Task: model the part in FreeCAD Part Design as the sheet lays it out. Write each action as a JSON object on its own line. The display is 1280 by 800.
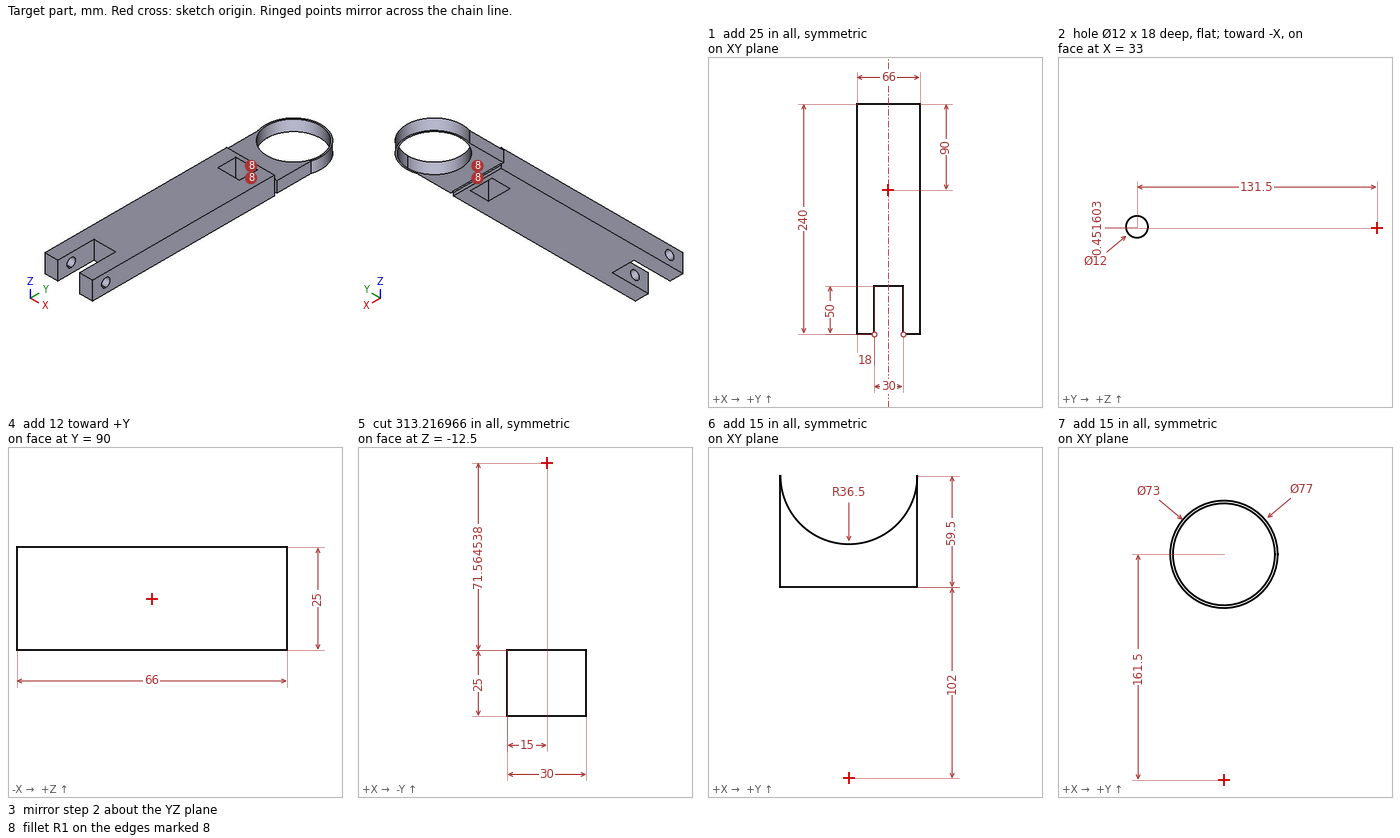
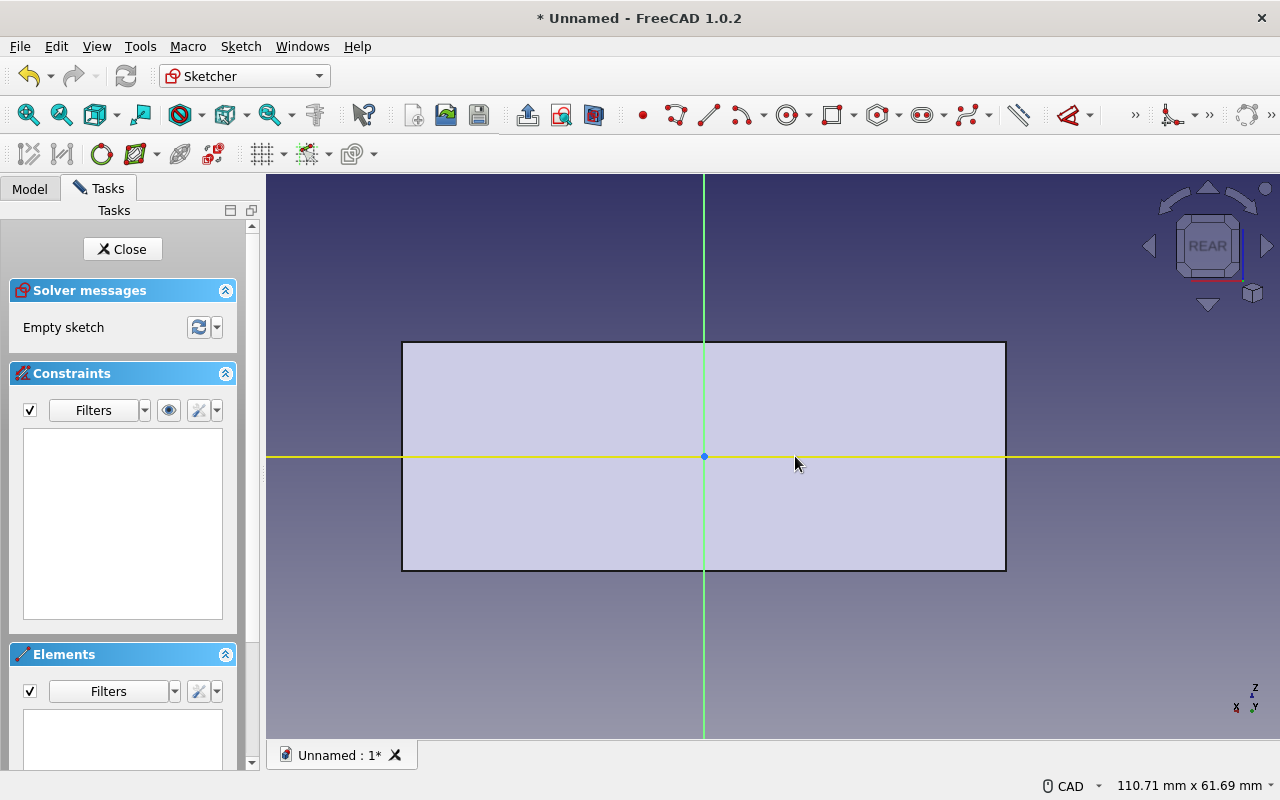
{"action": "left_click", "coordinate": [854, 116]}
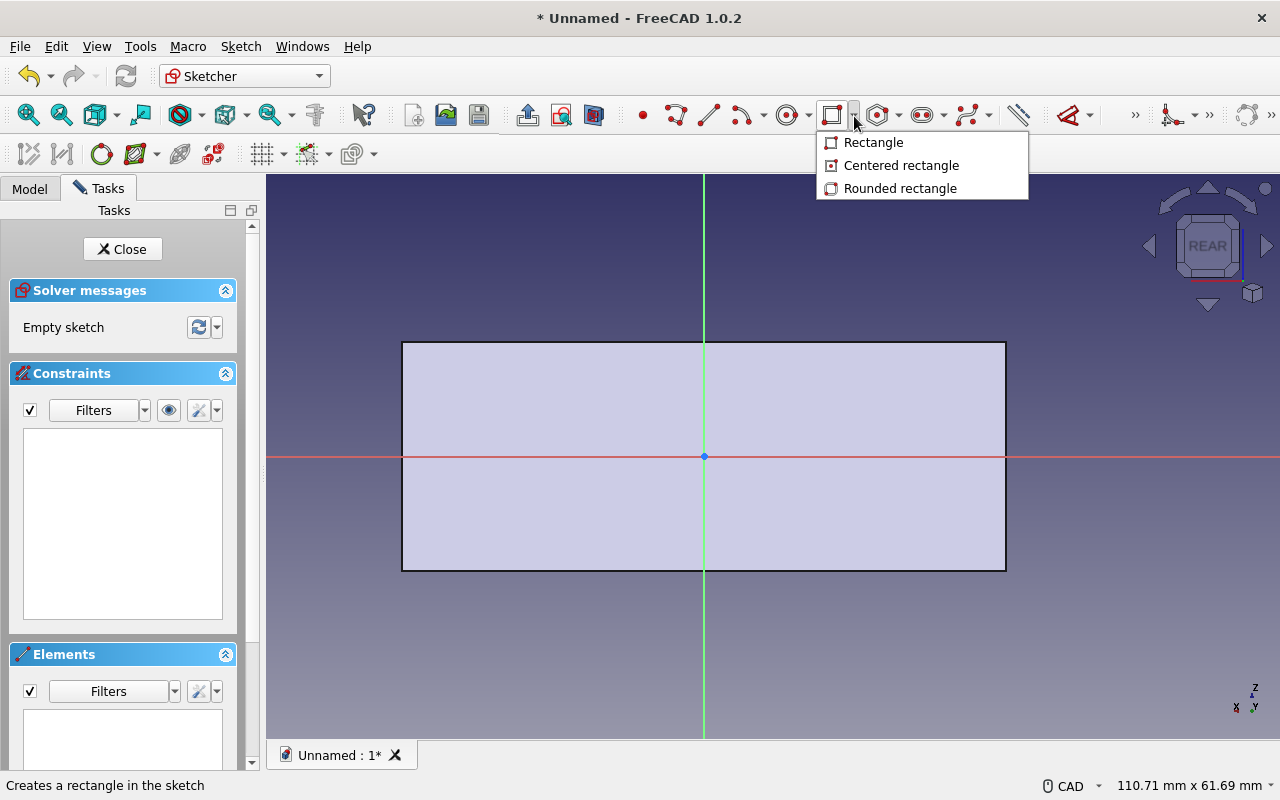
{"action": "left_click", "coordinate": [922, 166]}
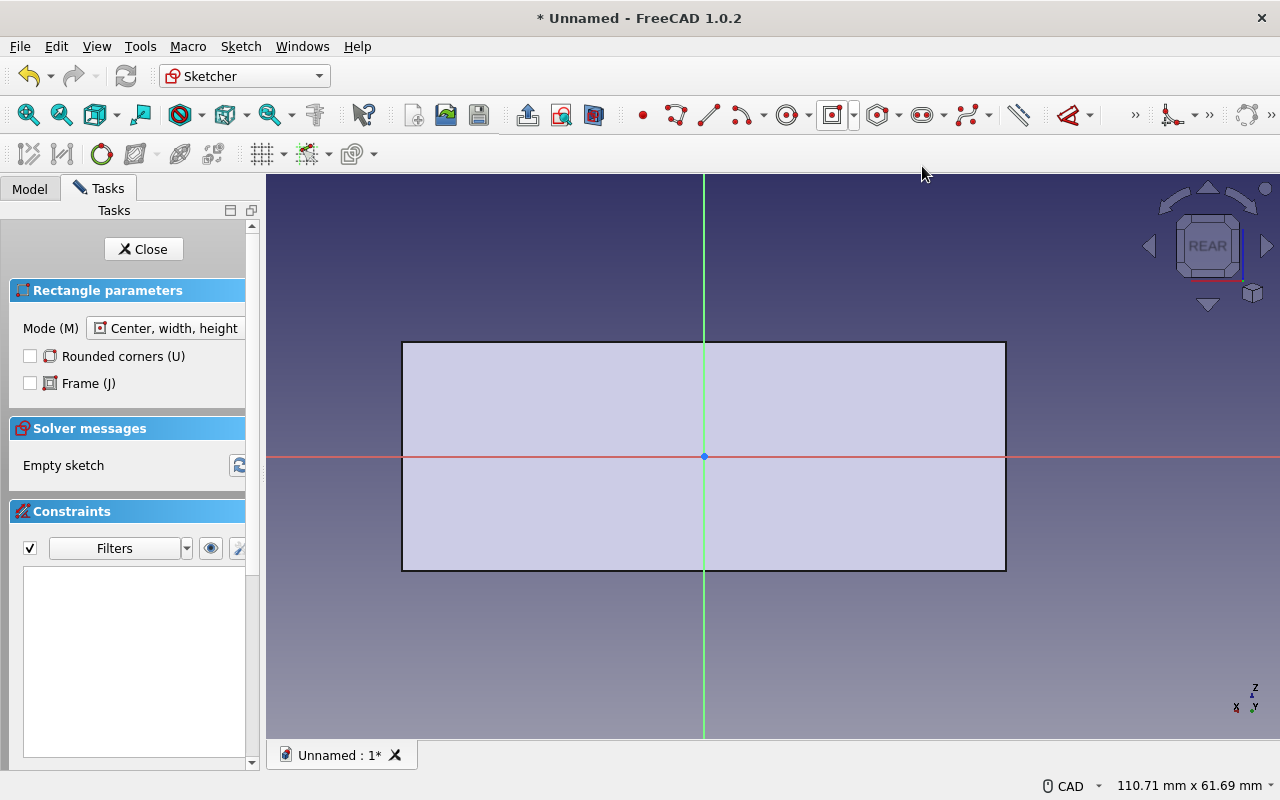
{"action": "left_click", "coordinate": [704, 456]}
{"action": "left_click", "coordinate": [1006, 342]}
{"action": "key", "text": "Escape"}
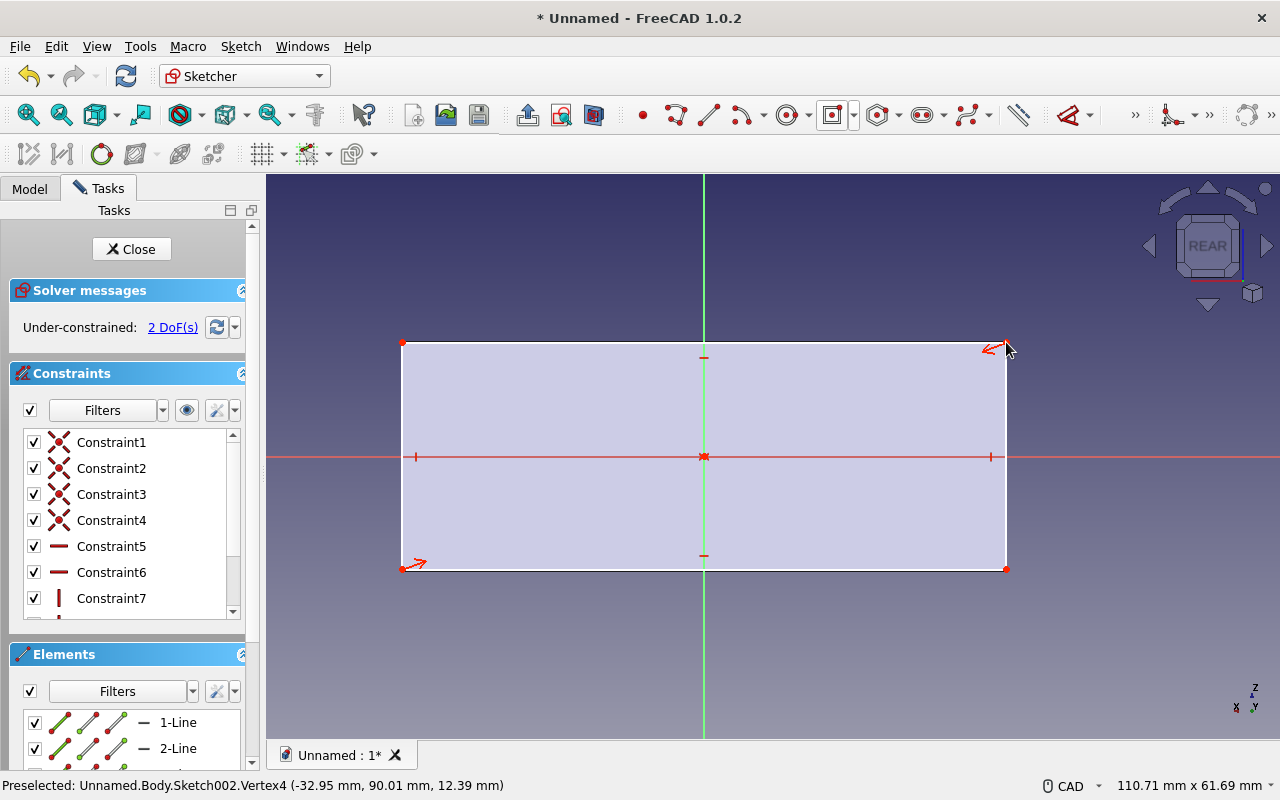
{"action": "key", "text": "d"}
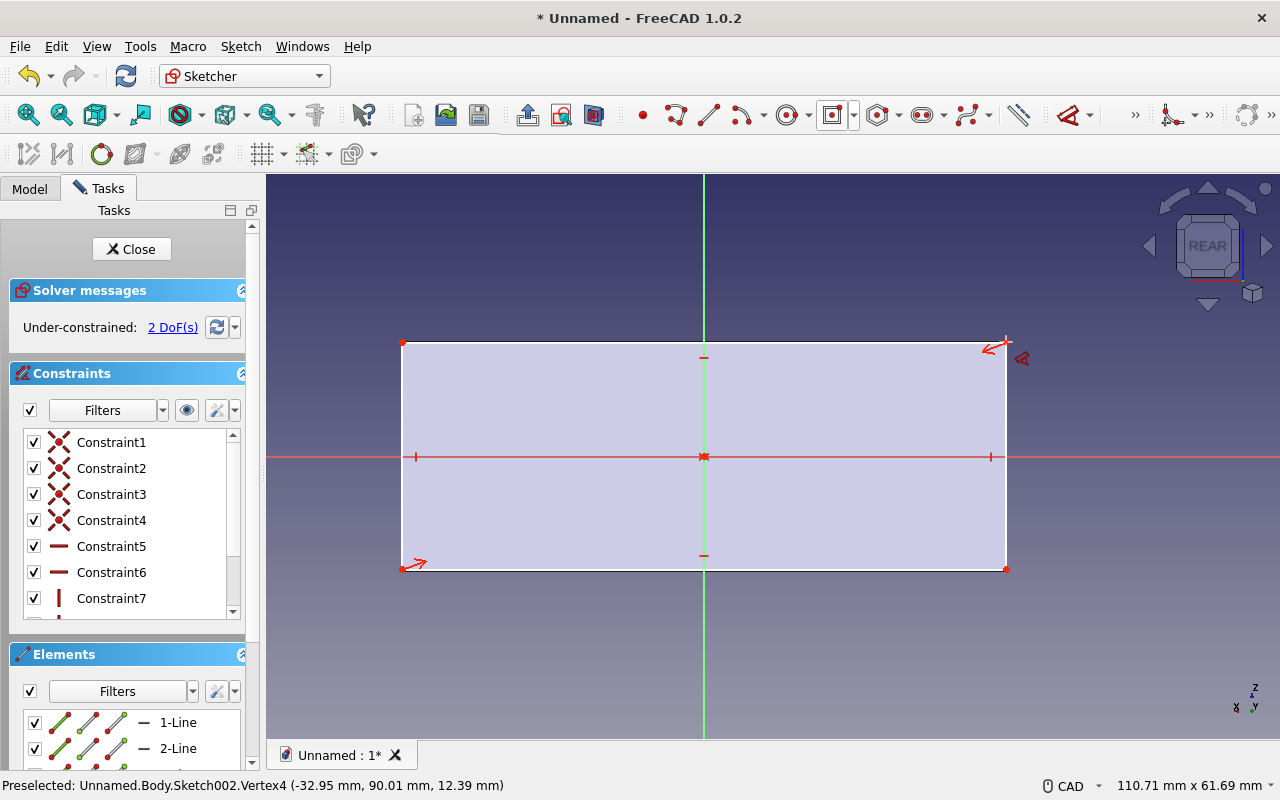
{"action": "left_click", "coordinate": [583, 570]}
{"action": "left_click", "coordinate": [565, 604]}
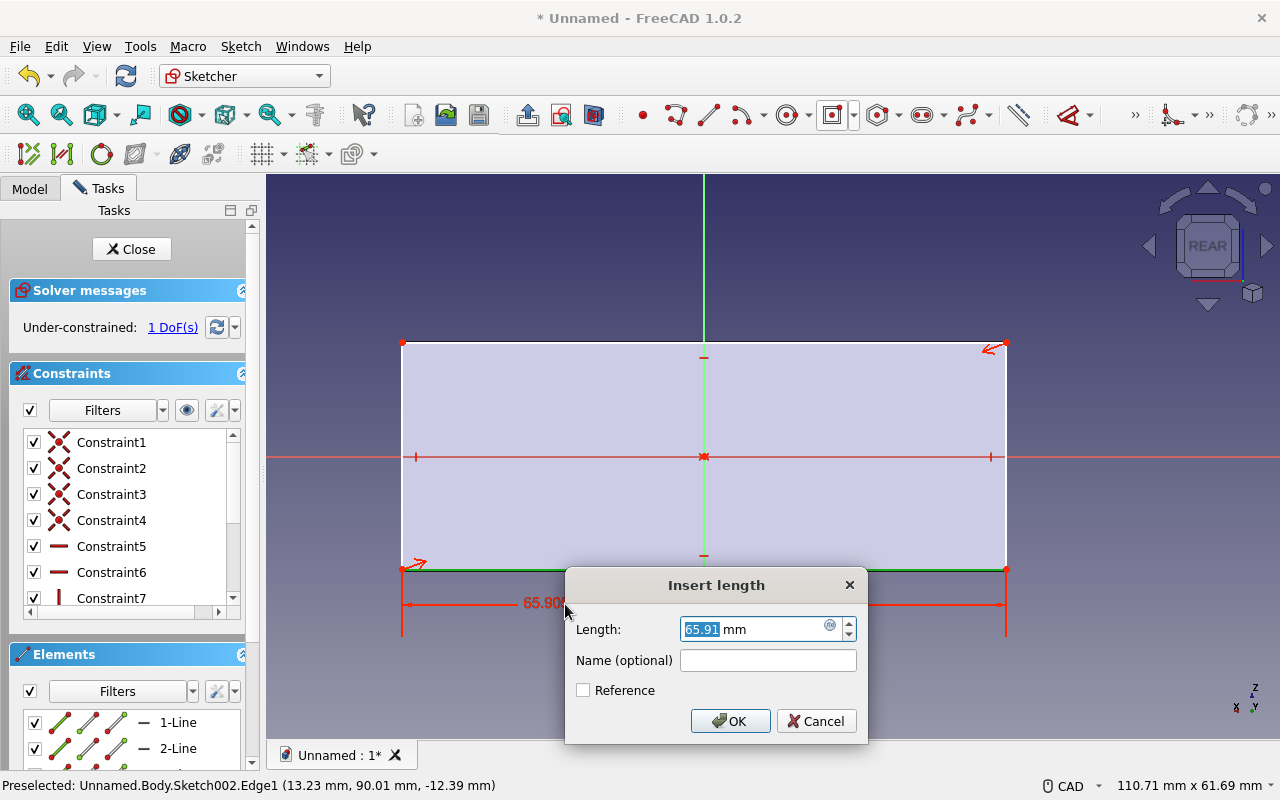
{"action": "type", "text": "66"}
{"action": "key", "text": "Return"}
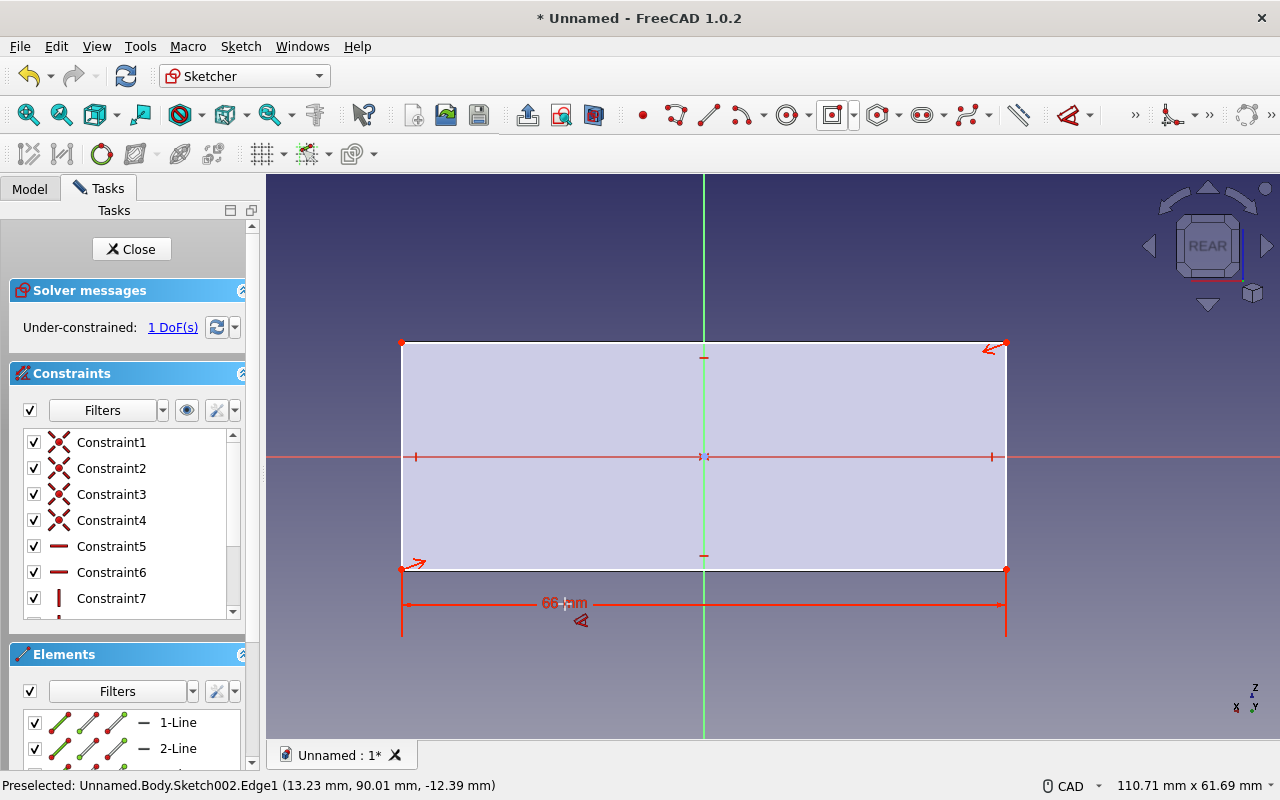
{"action": "left_click", "coordinate": [1006, 502]}
{"action": "left_click", "coordinate": [1040, 404]}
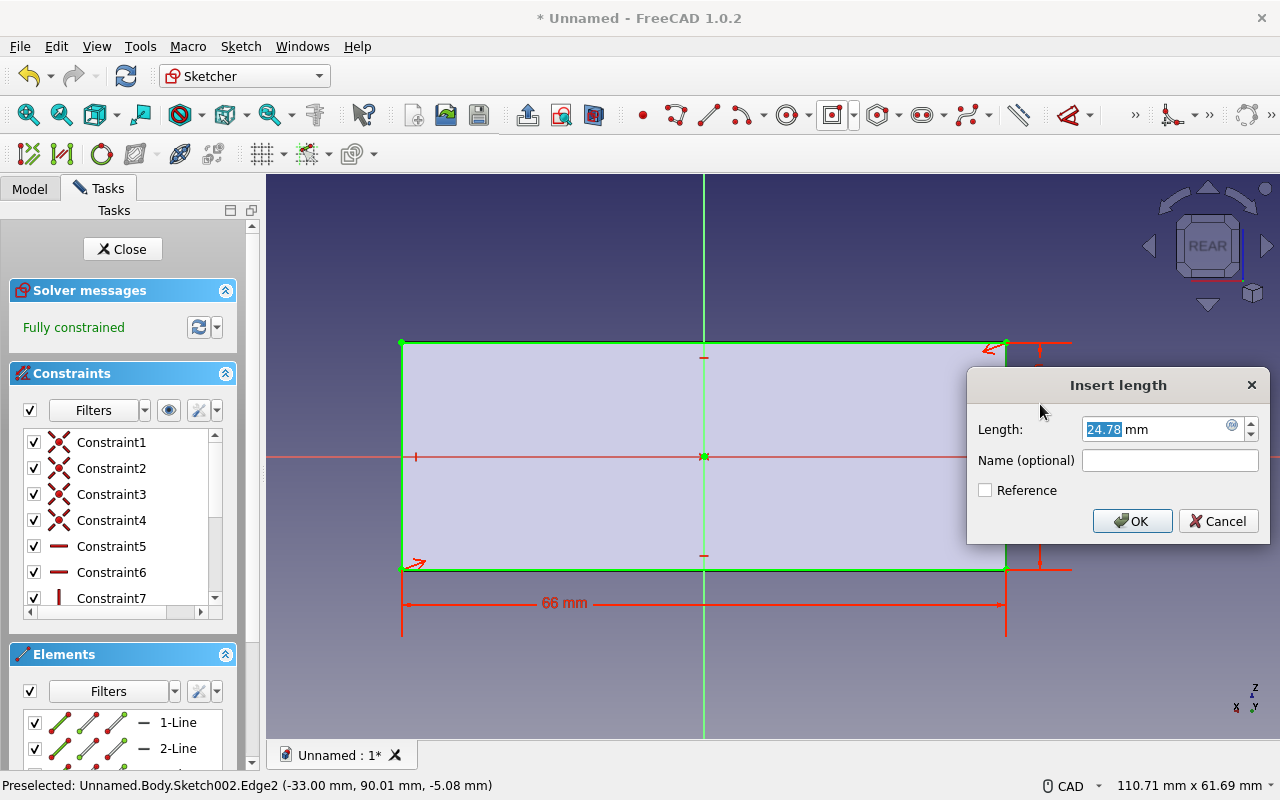
{"action": "type", "text": "25"}
{"action": "key", "text": "Return"}
{"action": "key", "text": "Escape"}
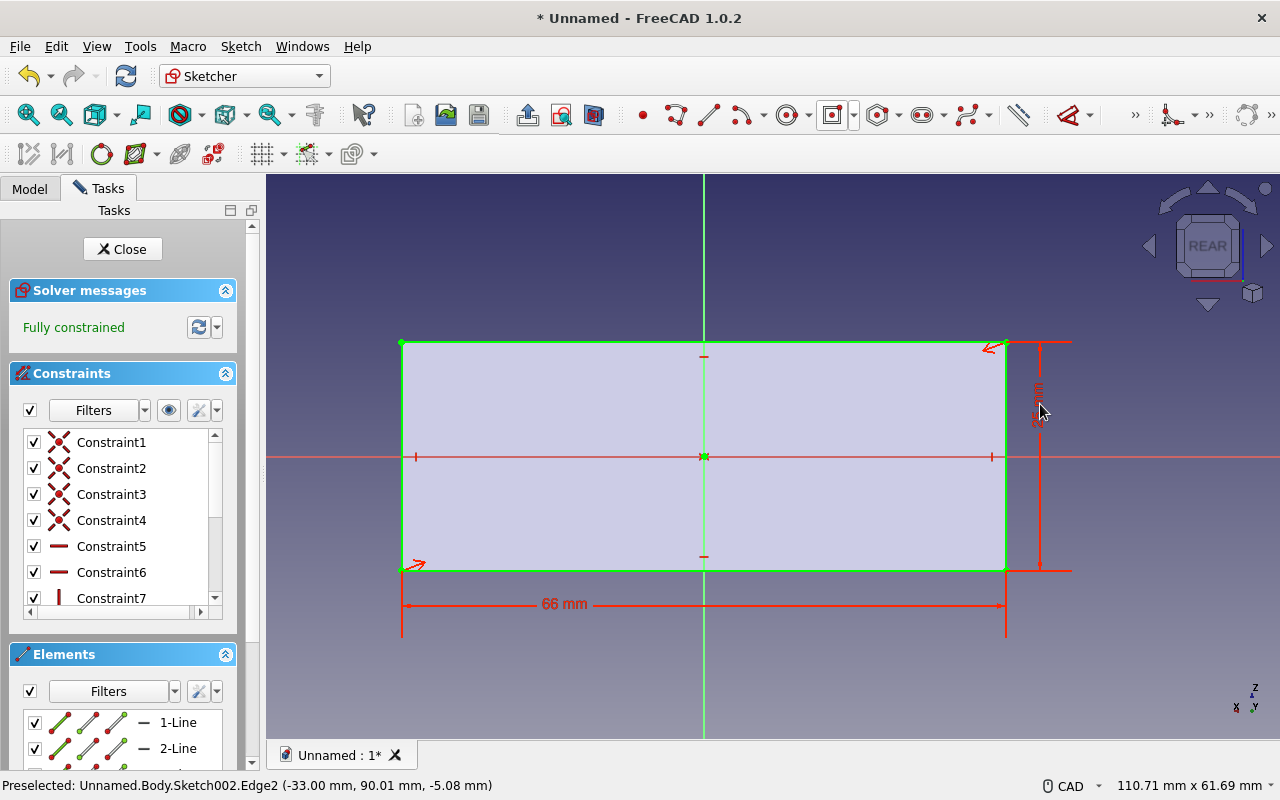
{"action": "left_click", "coordinate": [123, 249]}